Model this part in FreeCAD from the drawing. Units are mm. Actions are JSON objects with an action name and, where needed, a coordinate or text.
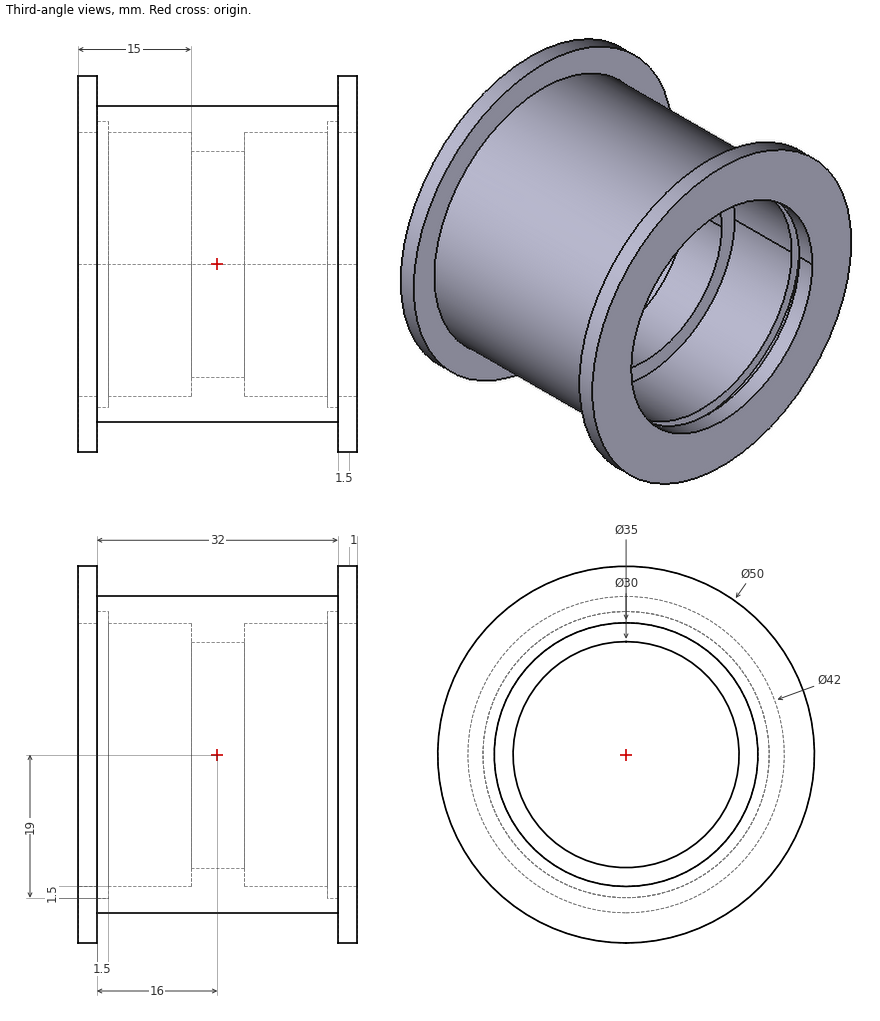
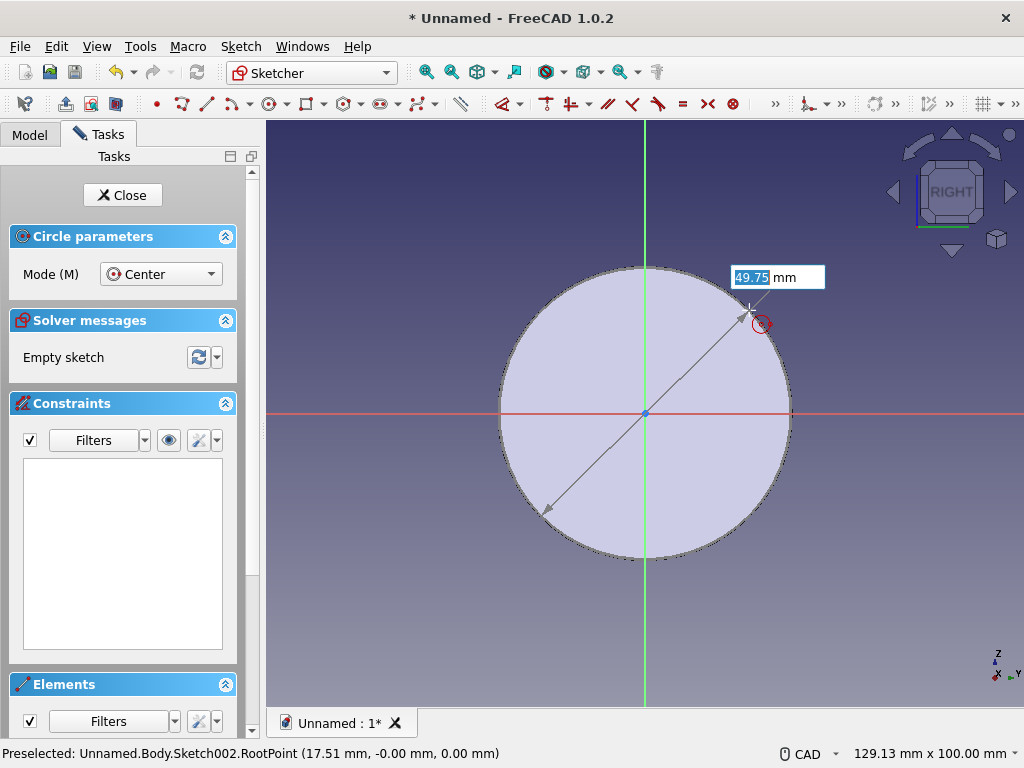
{"action": "type", "text": "50"}
{"action": "key", "text": "Return"}
{"action": "key", "text": "Escape"}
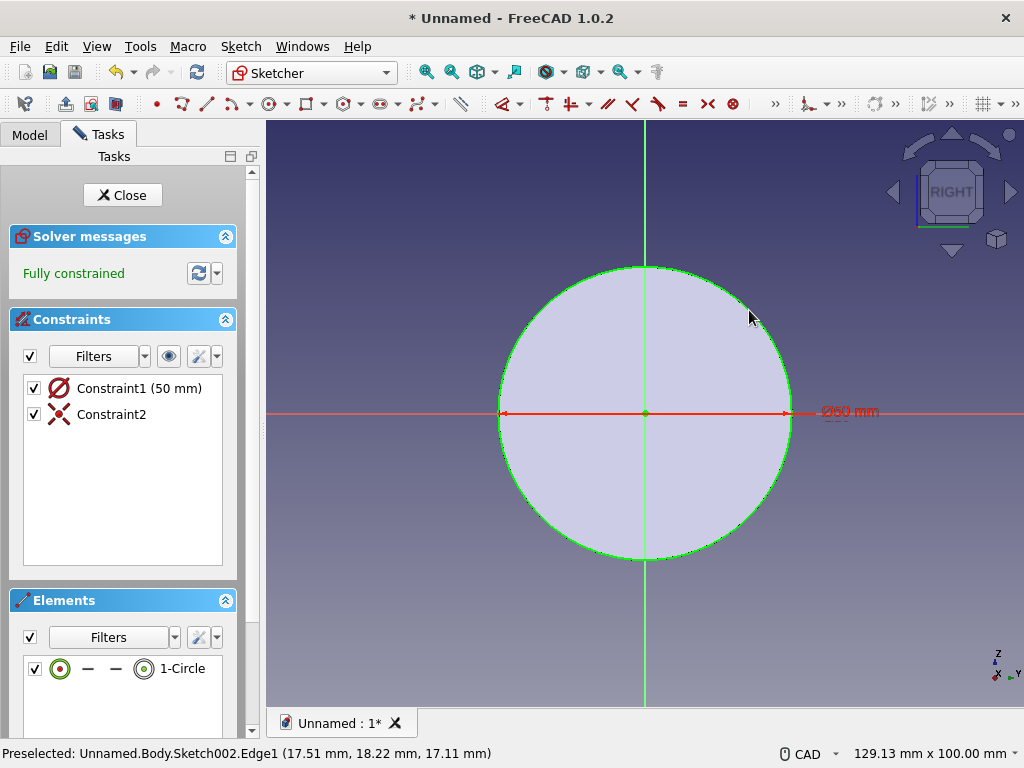
{"action": "left_click", "coordinate": [123, 195]}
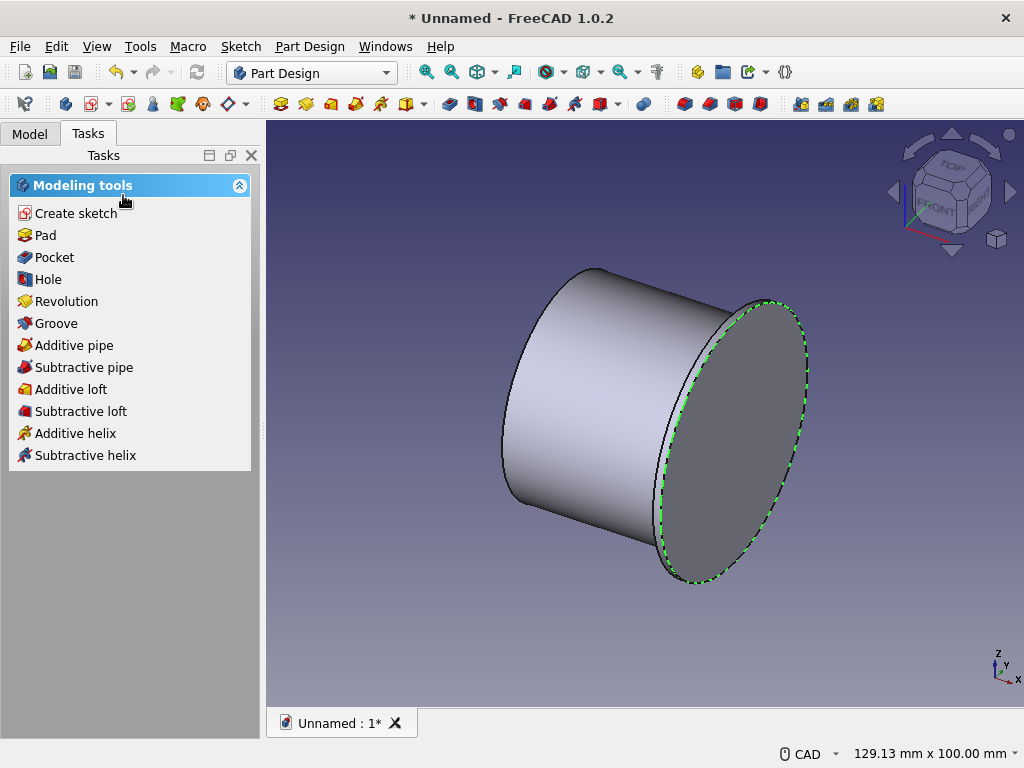
{"action": "left_click", "coordinate": [281, 104]}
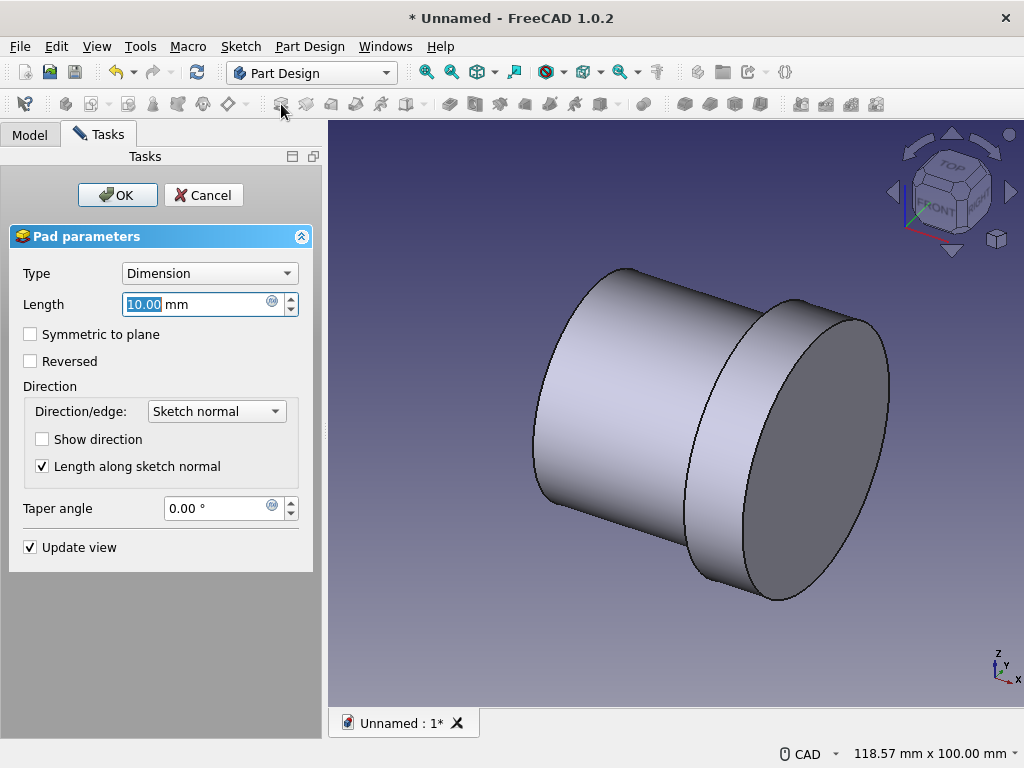
{"action": "type", "text": "1"}
{"action": "key", "text": "Tab"}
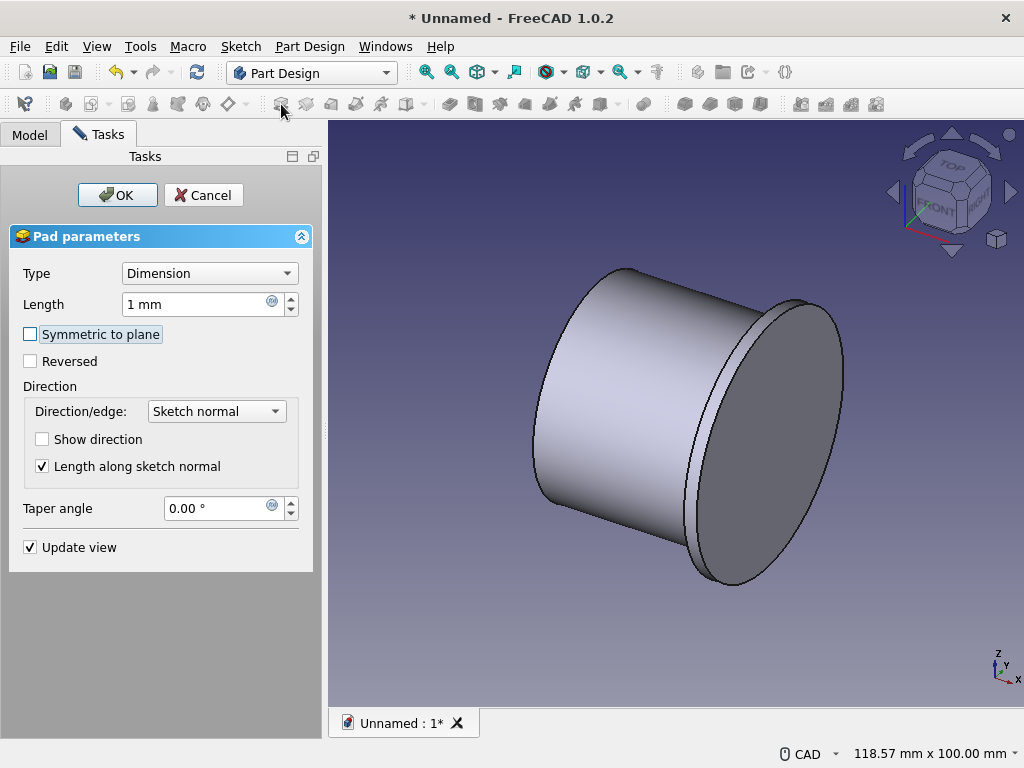
{"action": "left_click", "coordinate": [118, 195]}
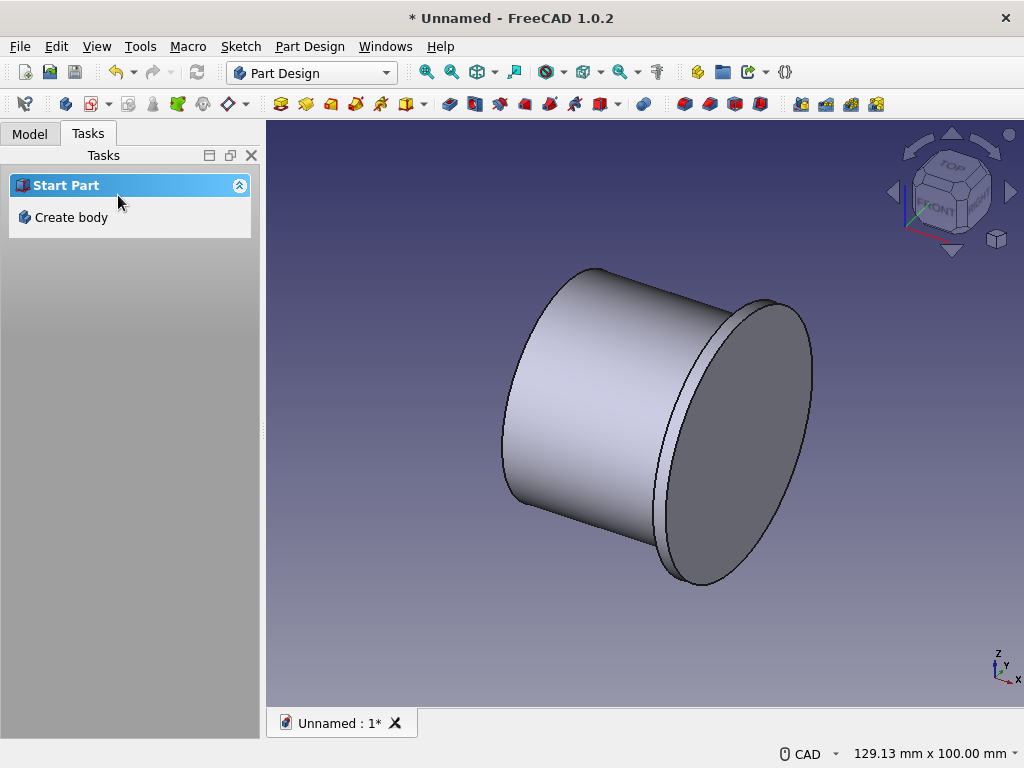
{"action": "left_click", "coordinate": [30, 134]}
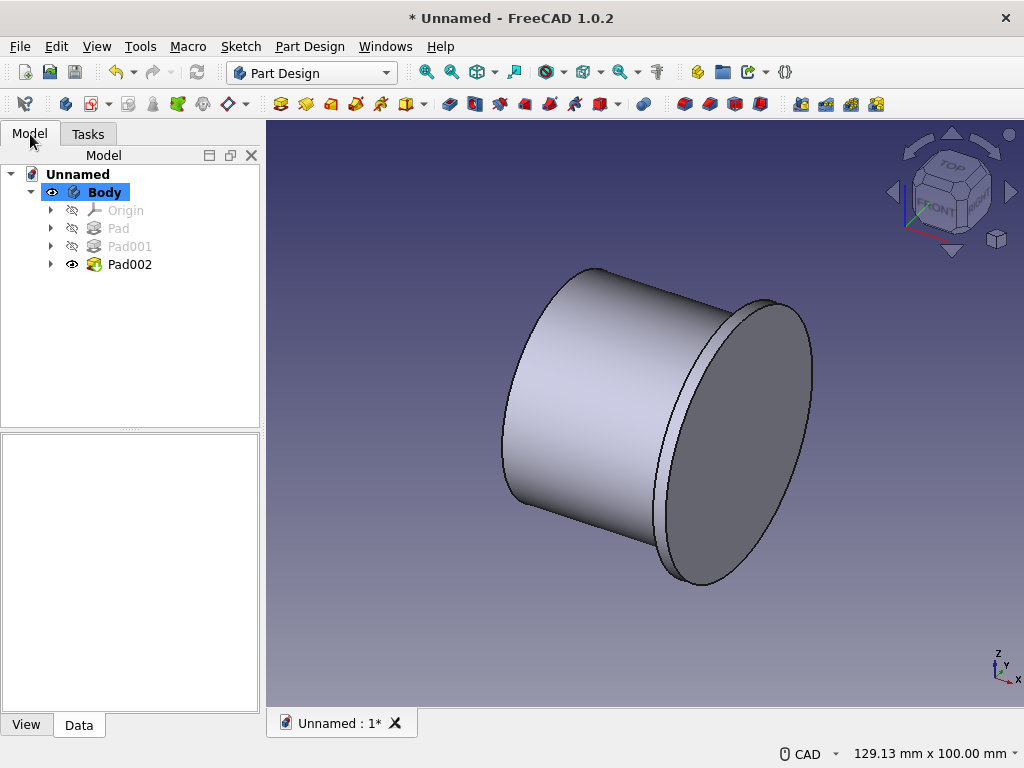
{"action": "left_click", "coordinate": [117, 246]}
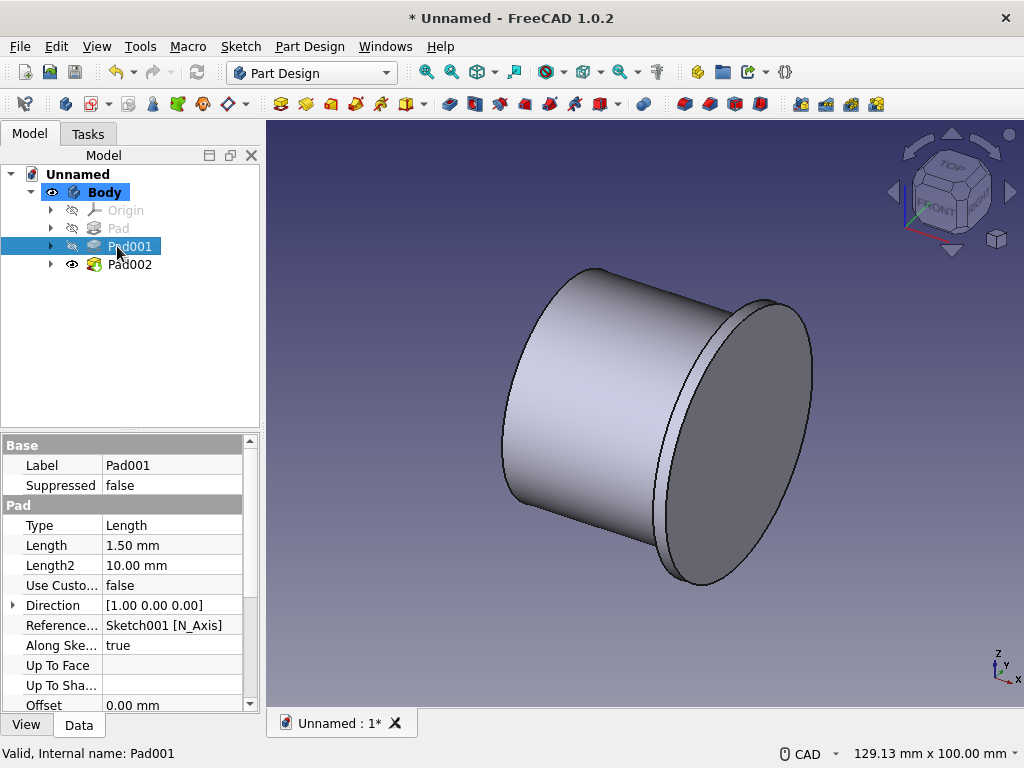
{"action": "left_click", "coordinate": [117, 264], "text": "ctrl"}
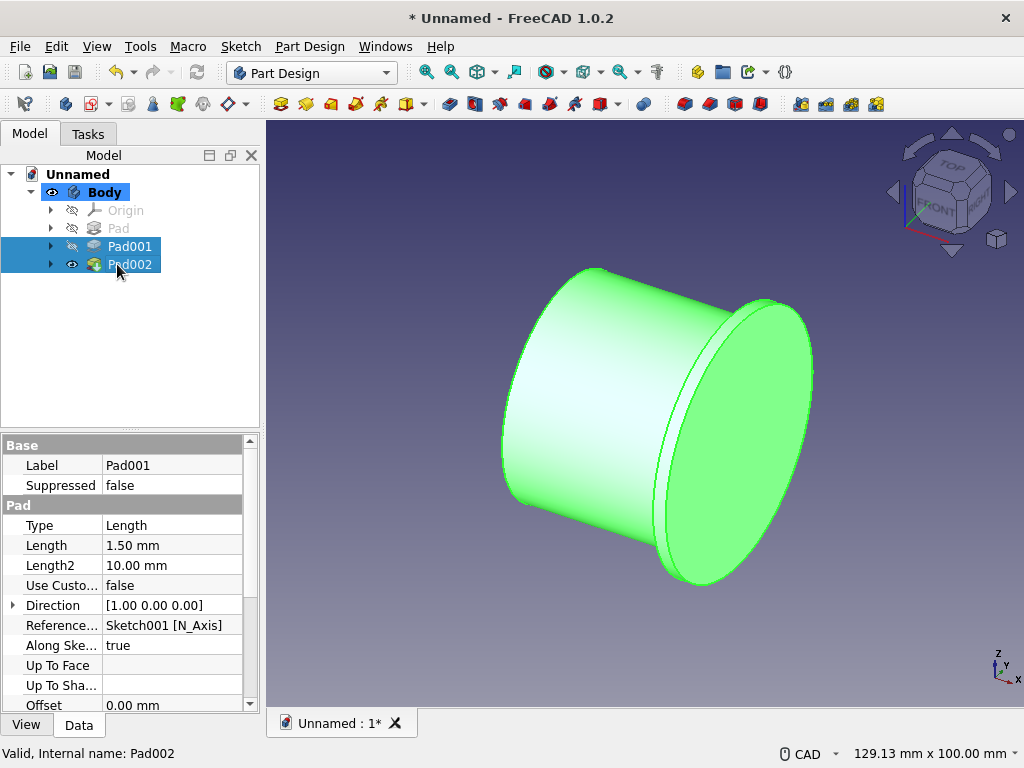
{"action": "left_click", "coordinate": [801, 104]}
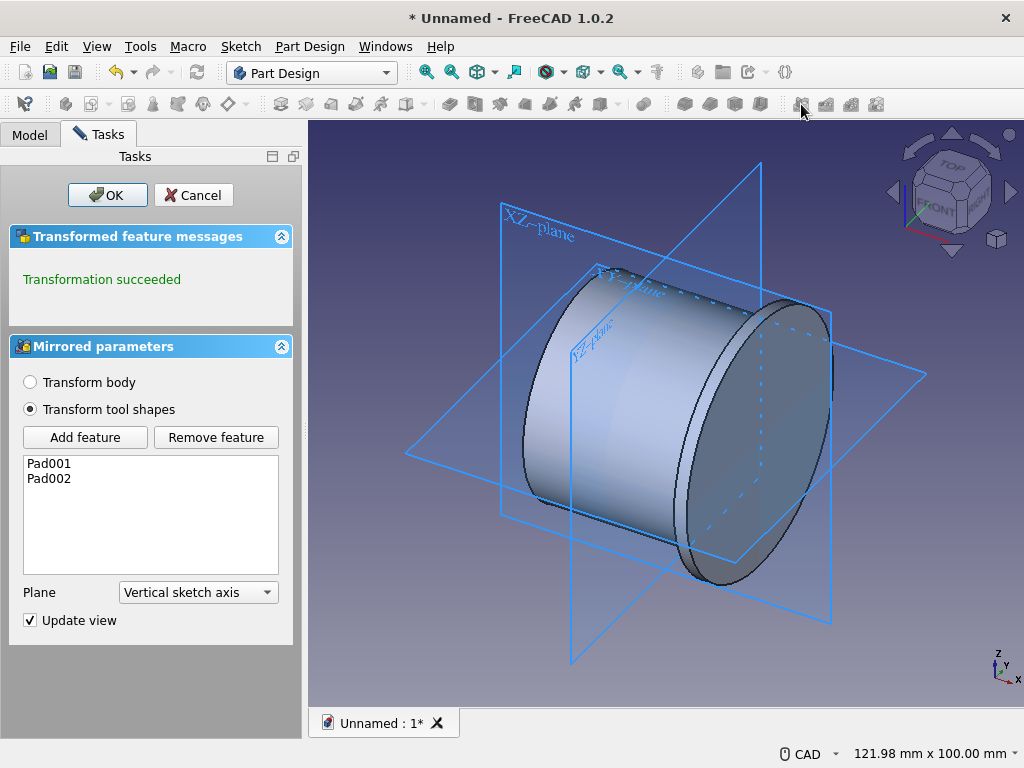
{"action": "left_click", "coordinate": [199, 592]}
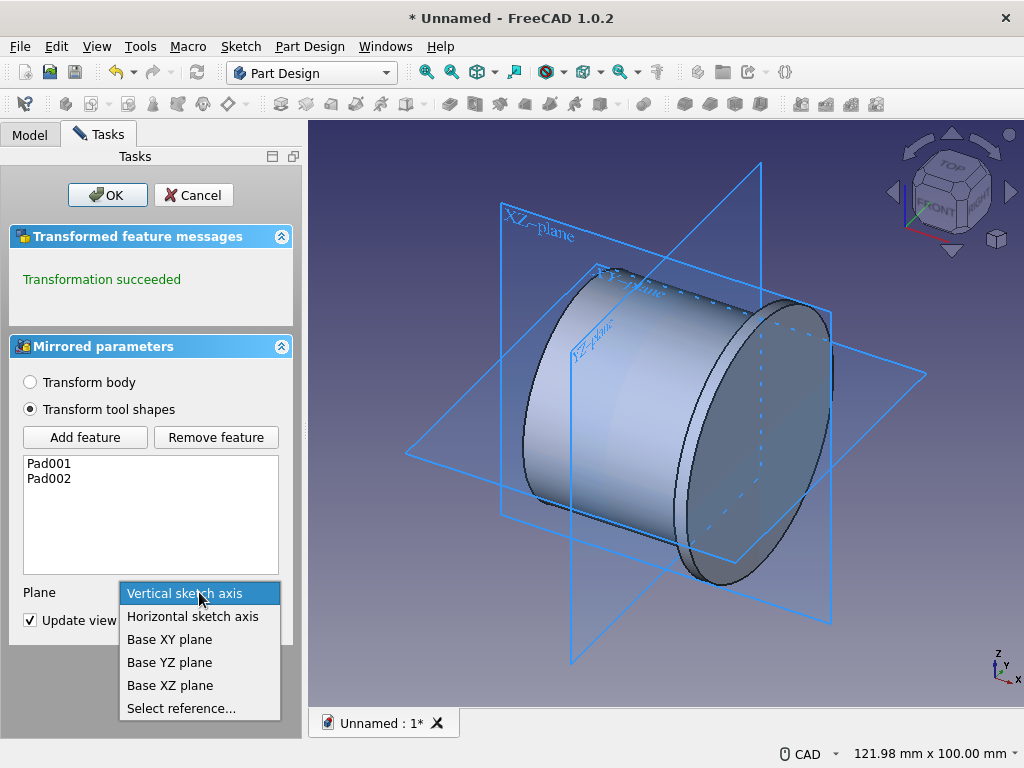
{"action": "left_click", "coordinate": [198, 662]}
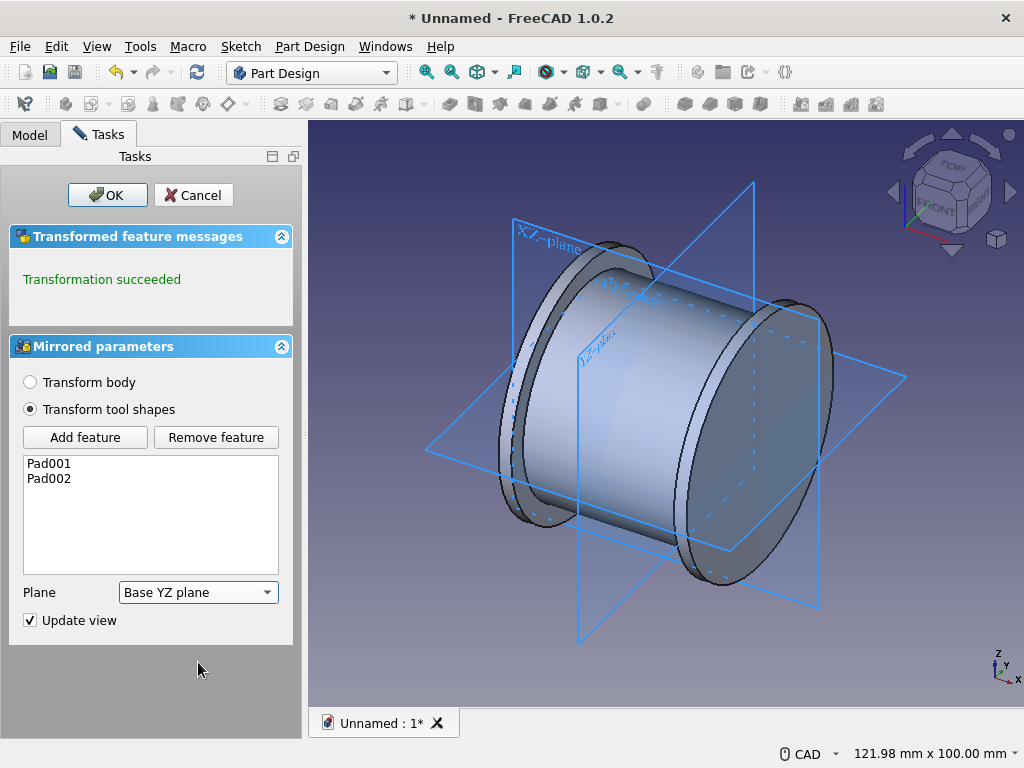
{"action": "left_click", "coordinate": [108, 195]}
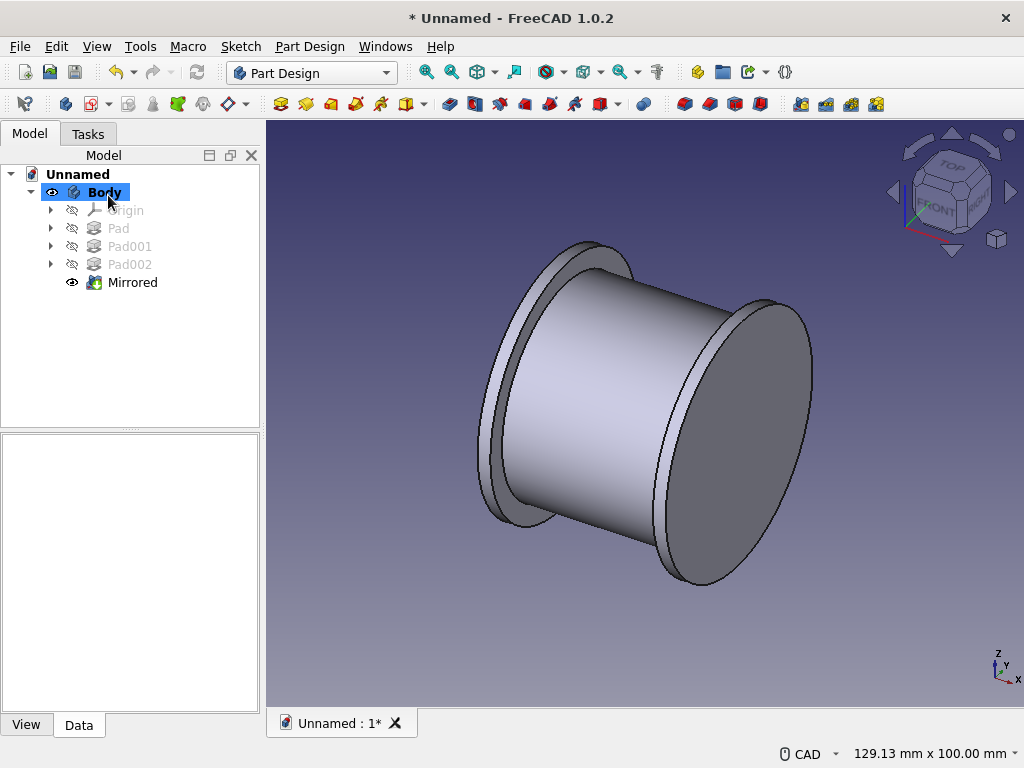
{"action": "key", "text": "6"}